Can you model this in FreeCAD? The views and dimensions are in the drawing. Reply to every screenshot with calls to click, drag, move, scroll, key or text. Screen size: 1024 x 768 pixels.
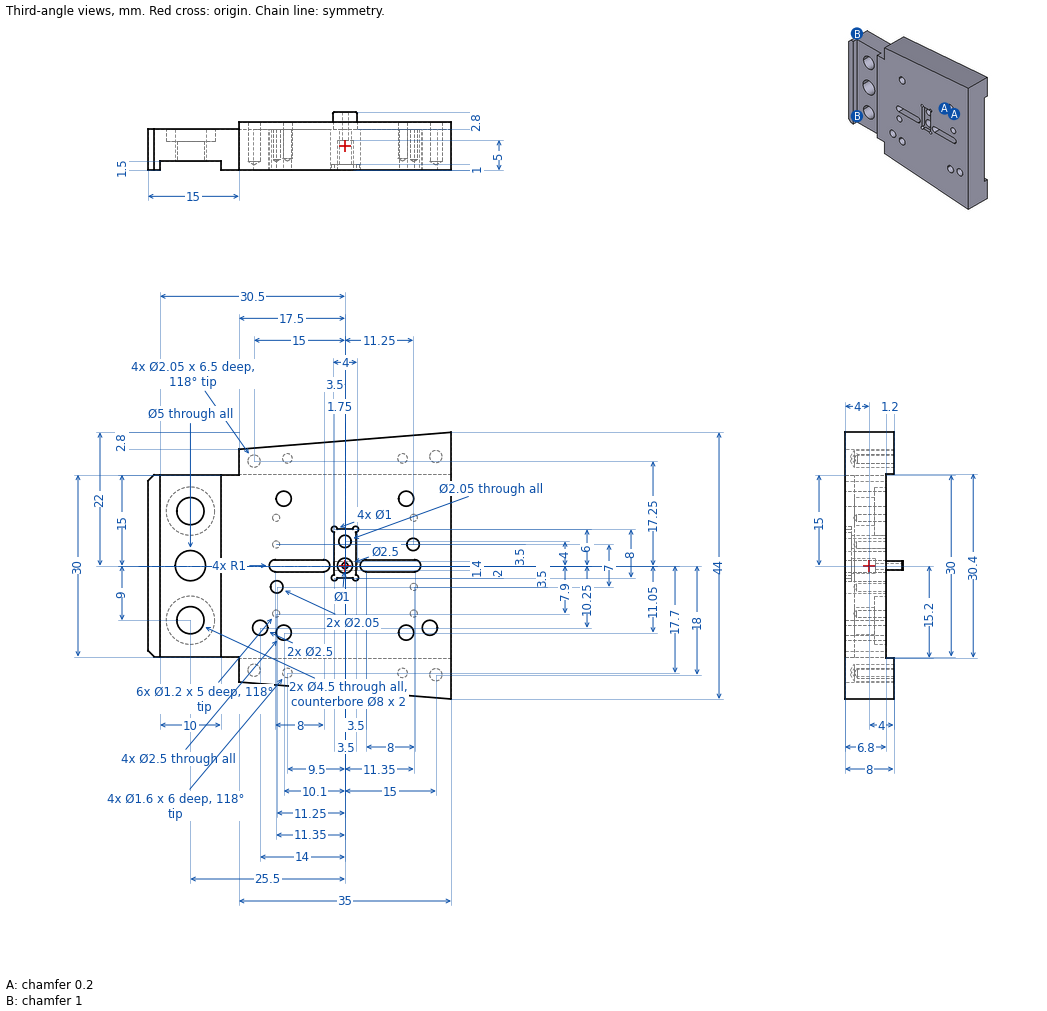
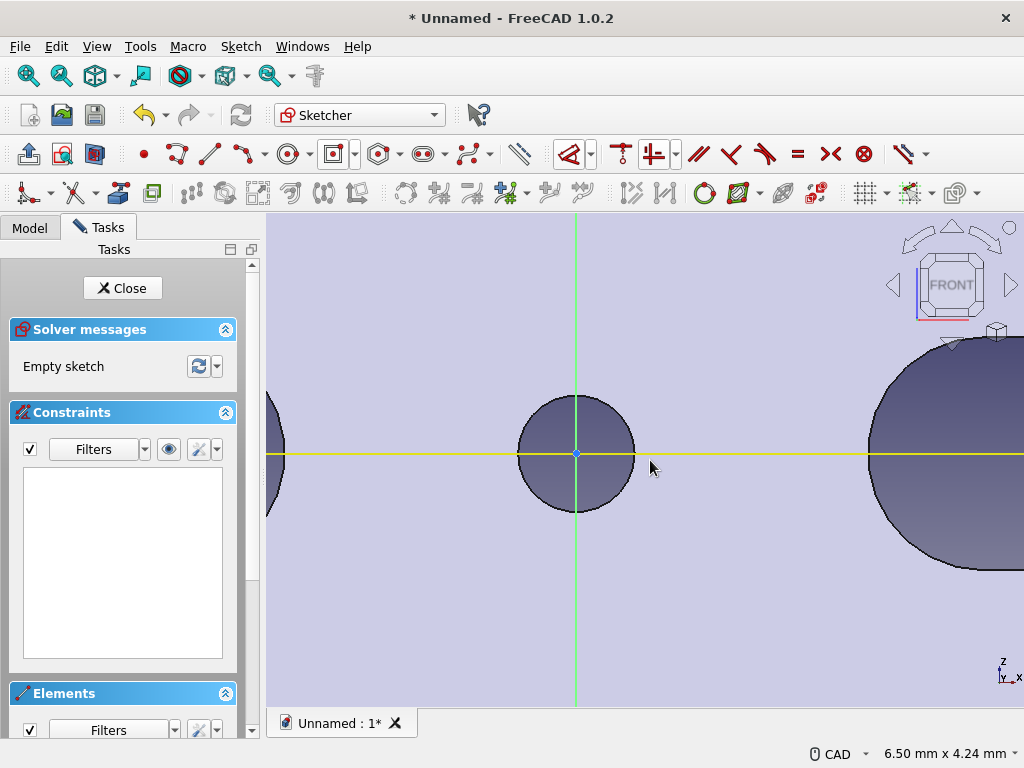
click(288, 154)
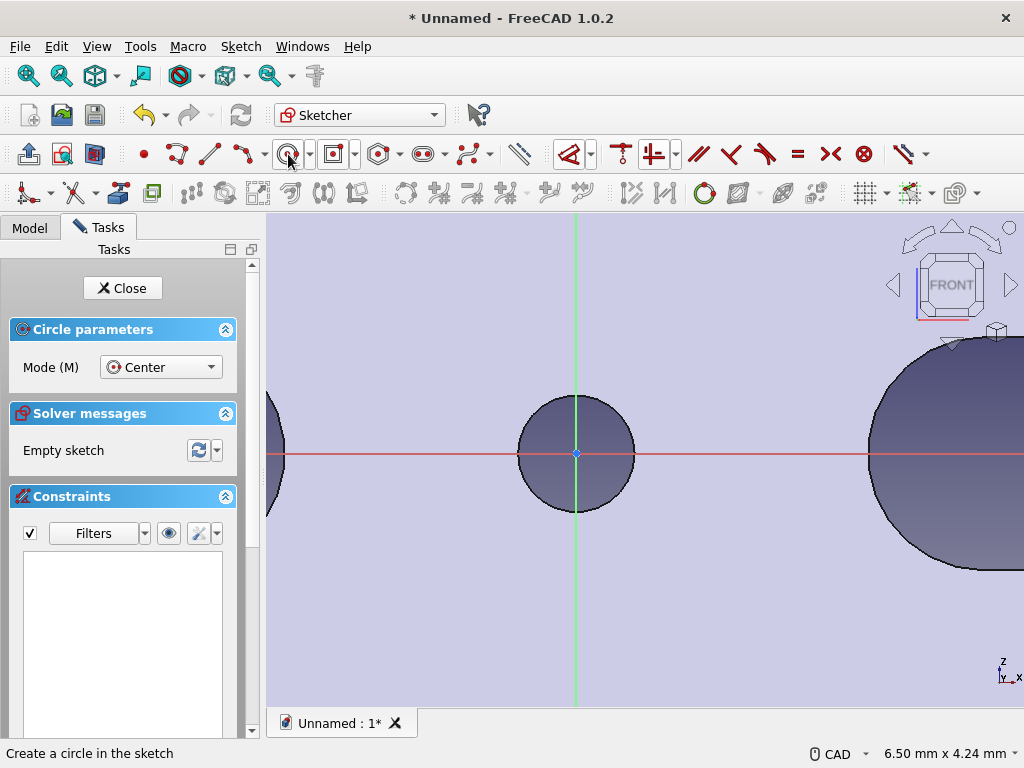
click(576, 454)
move(679, 351)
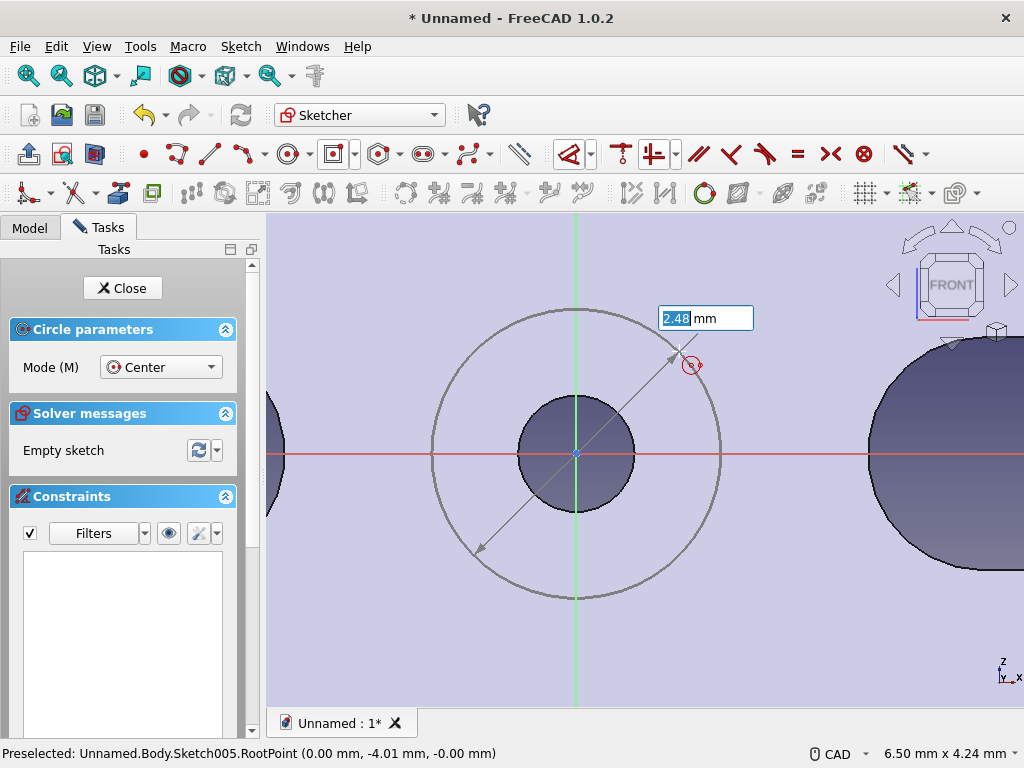
text(2.5)
key(Return)
key(Escape)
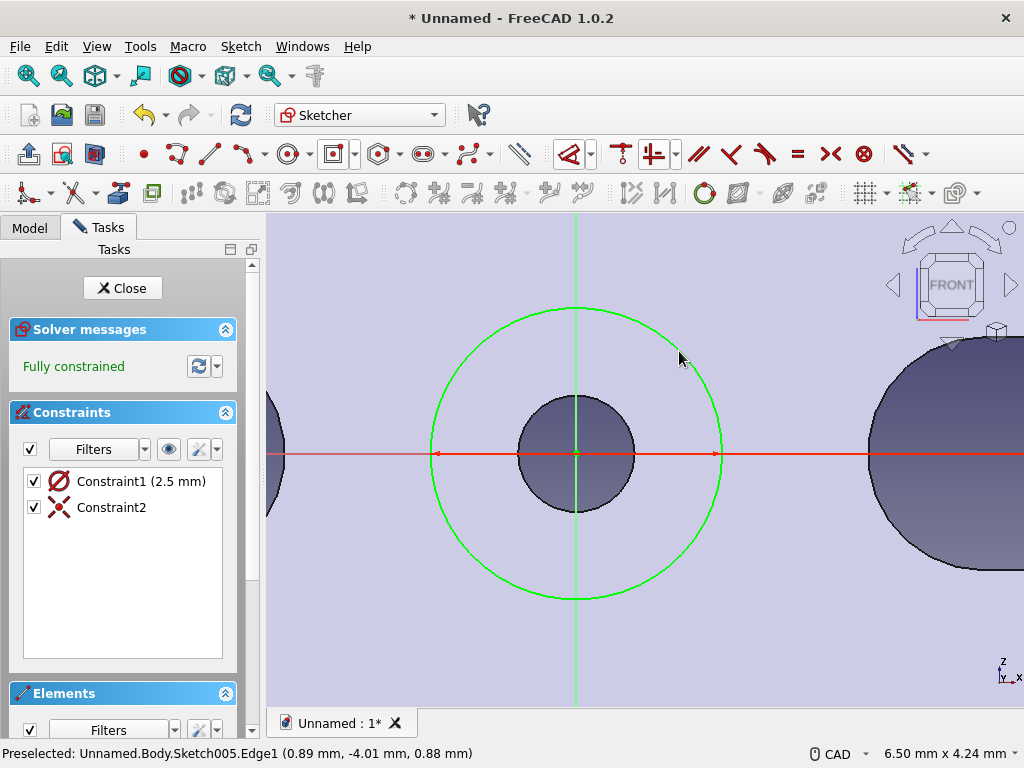
click(123, 288)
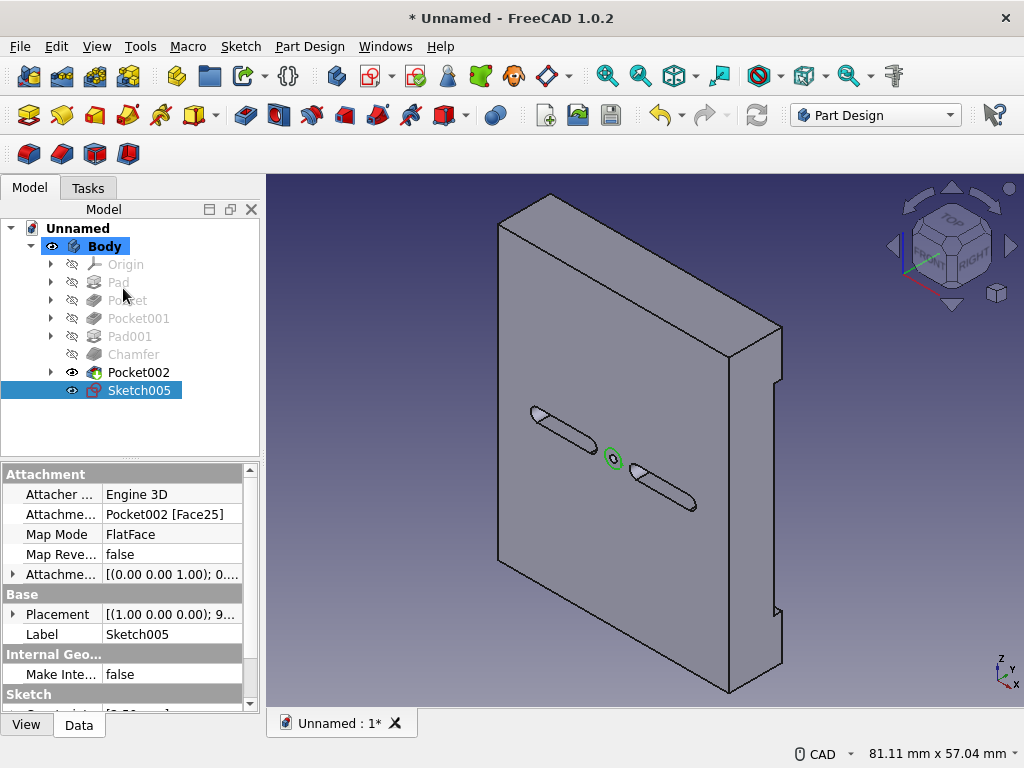
click(246, 116)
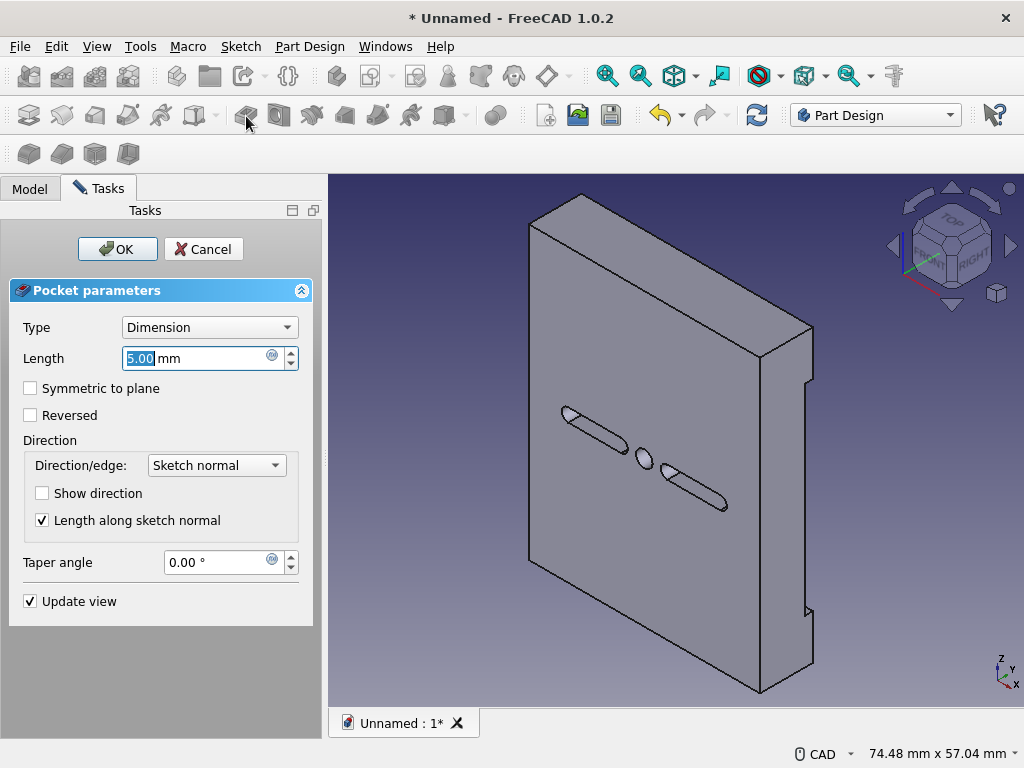
text(5)
key(Tab)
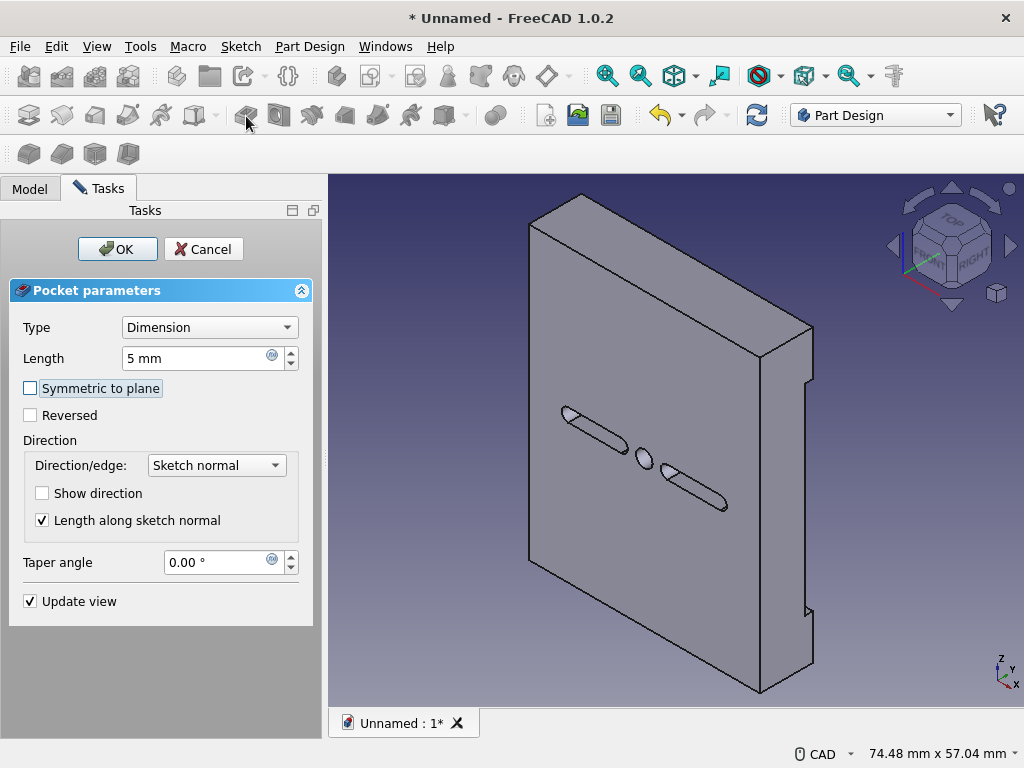
click(118, 249)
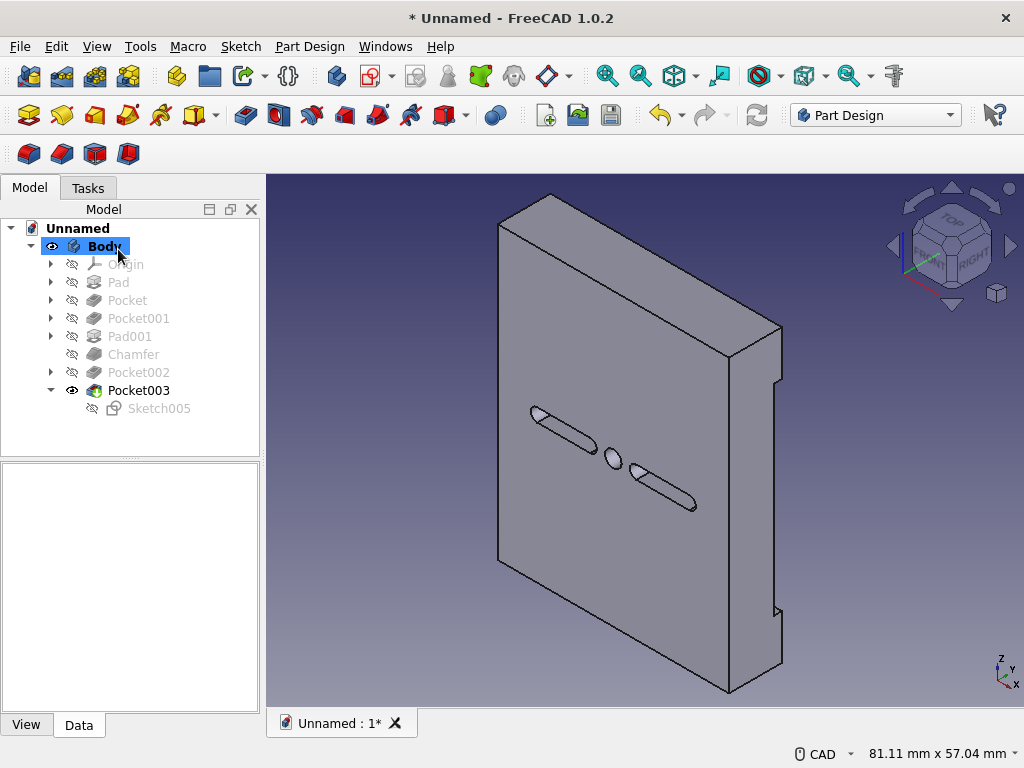
click(646, 573)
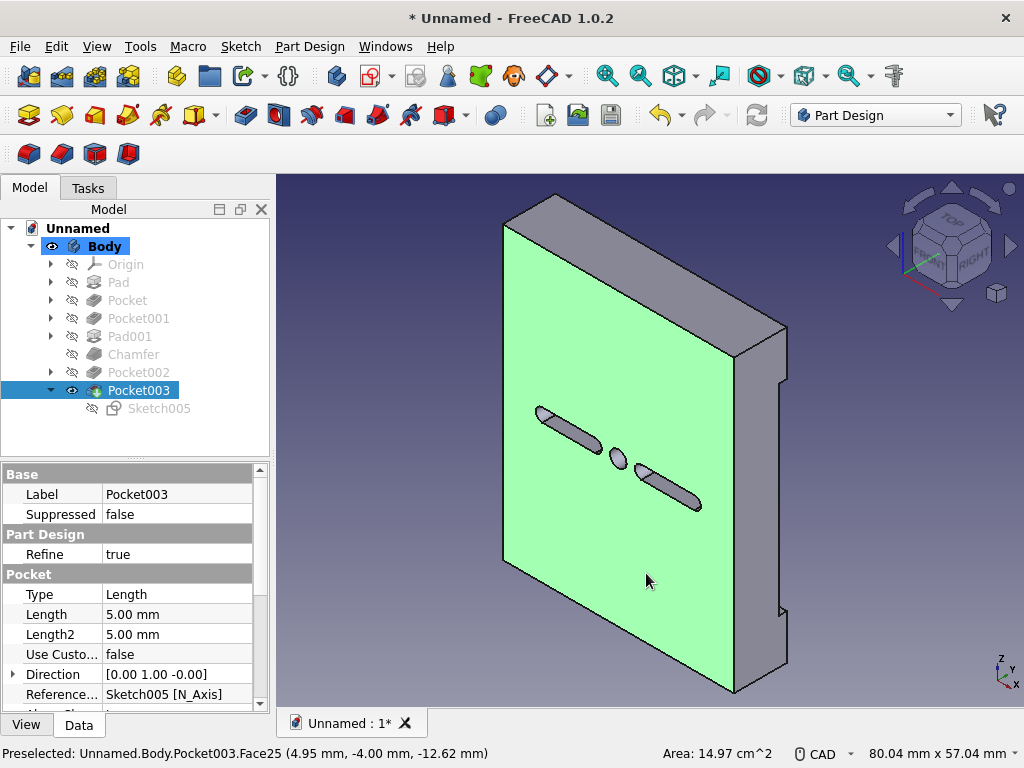
click(370, 76)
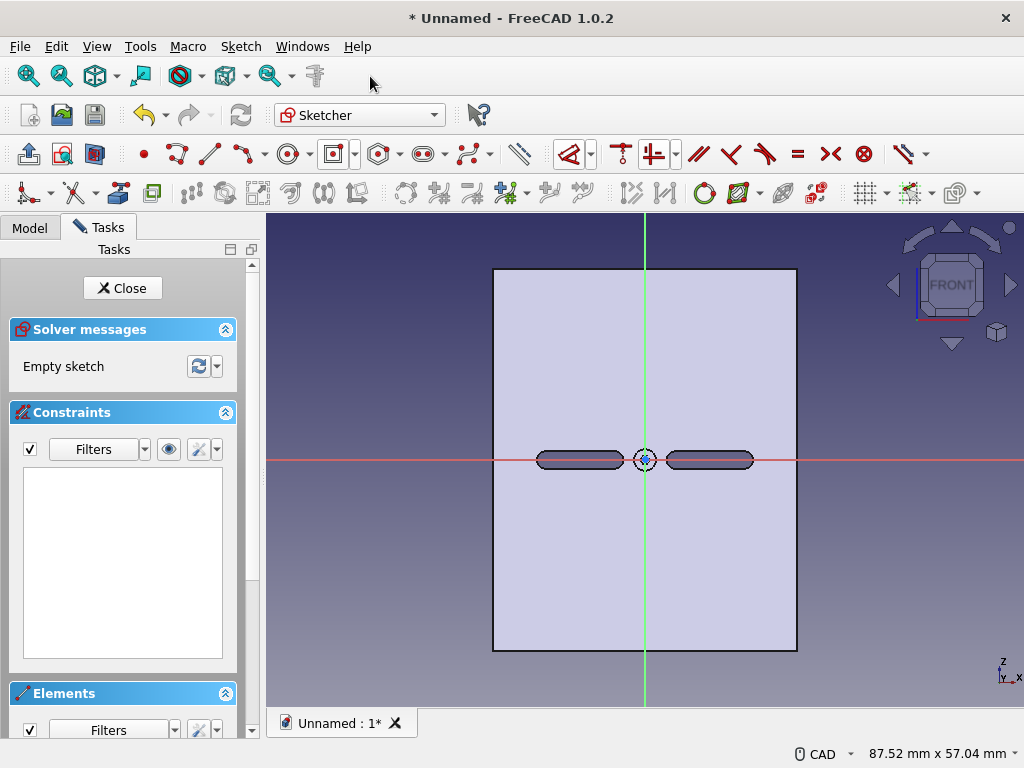
scroll(784, 611, up, 2)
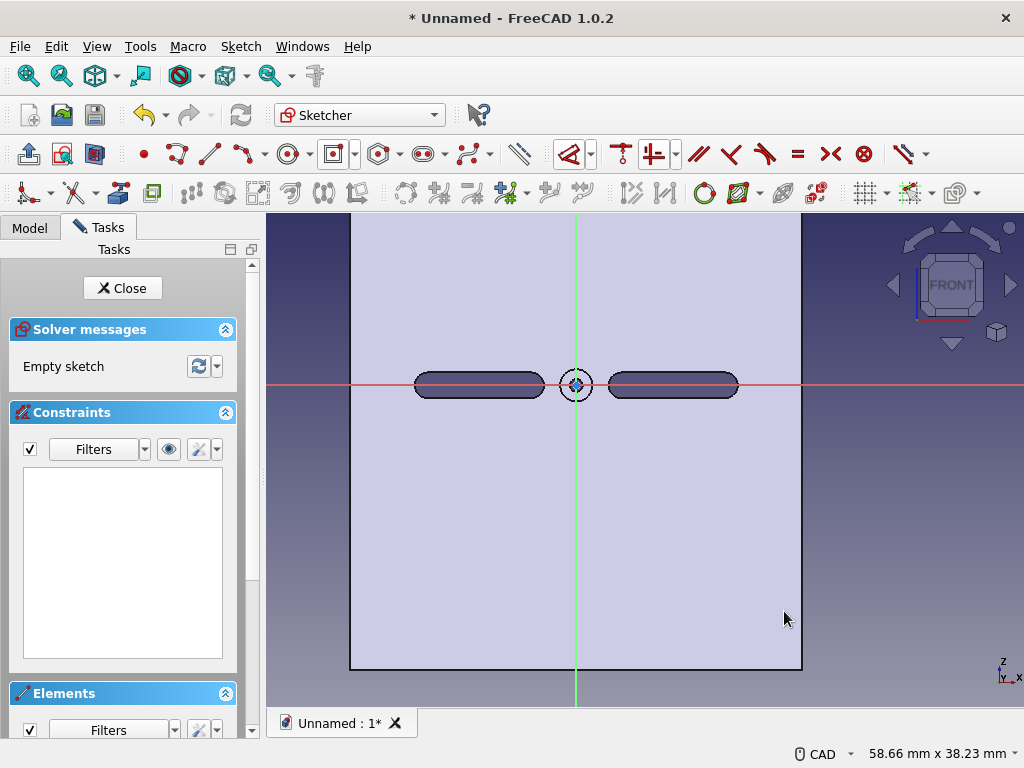
click(288, 154)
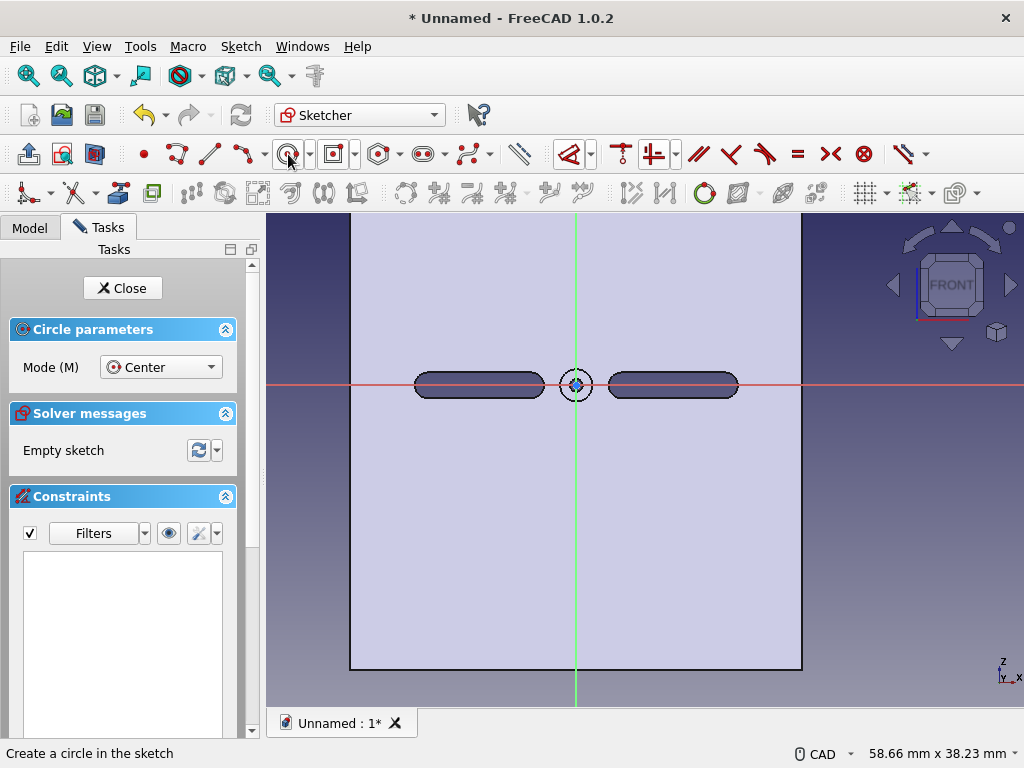
scroll(395, 518, up, 2)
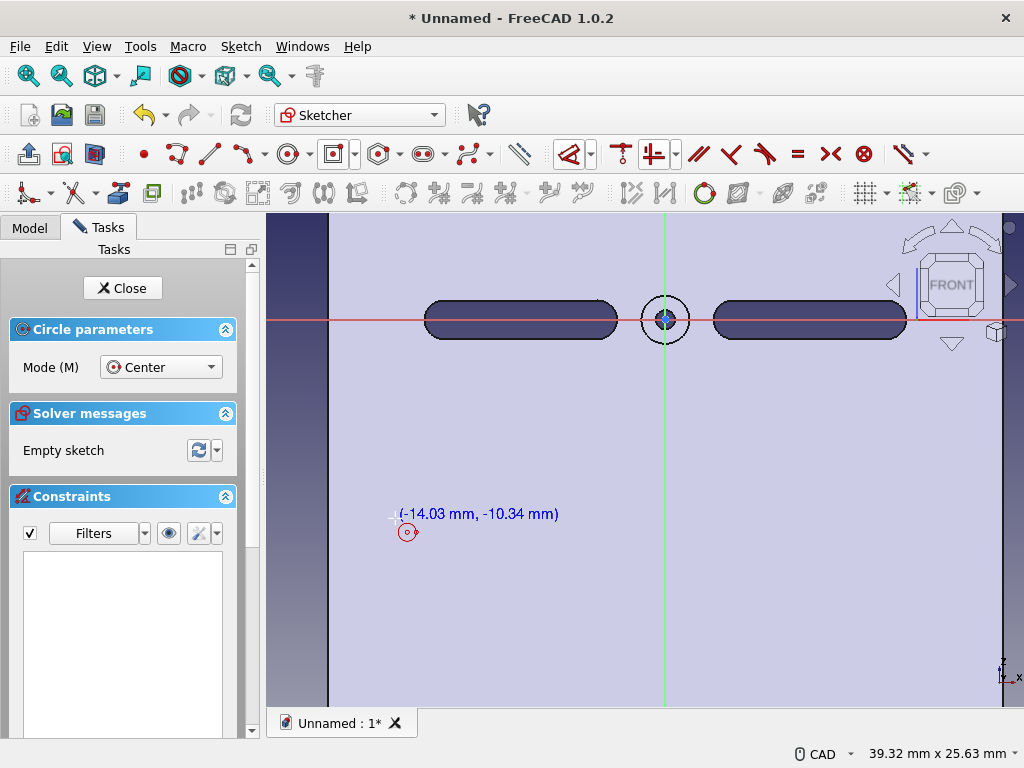
click(396, 517)
move(413, 500)